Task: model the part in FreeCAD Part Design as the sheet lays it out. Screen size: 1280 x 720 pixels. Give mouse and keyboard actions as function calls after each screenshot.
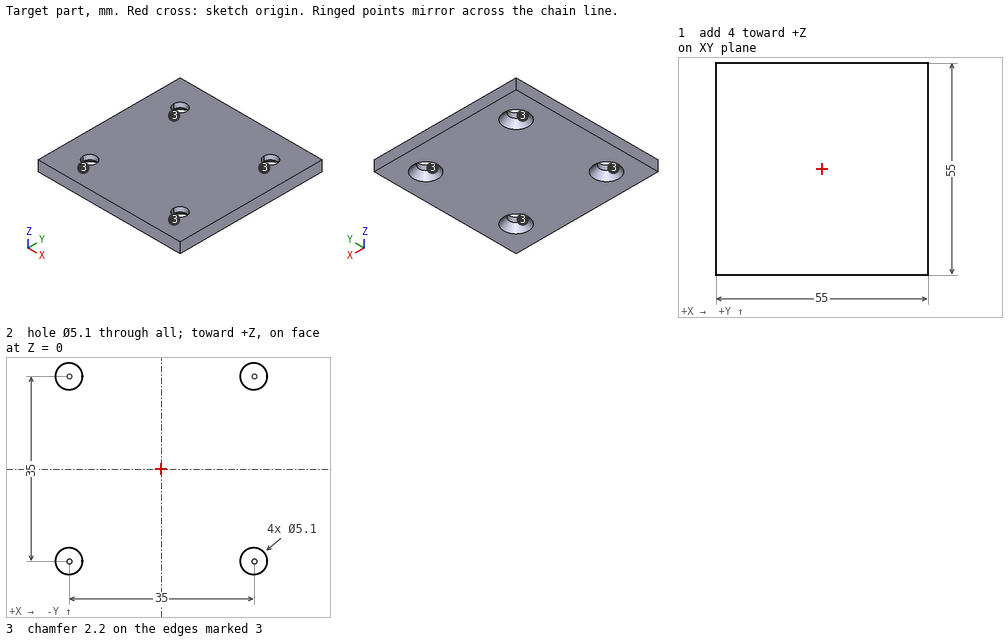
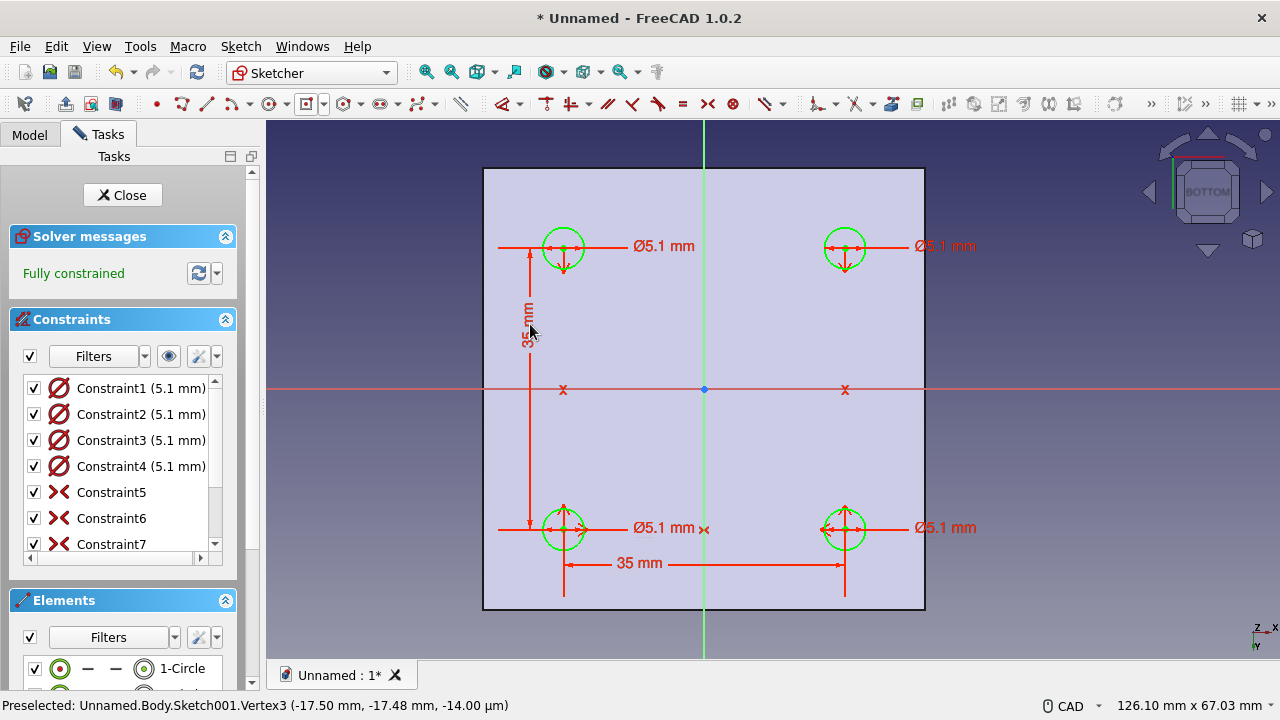
click(123, 195)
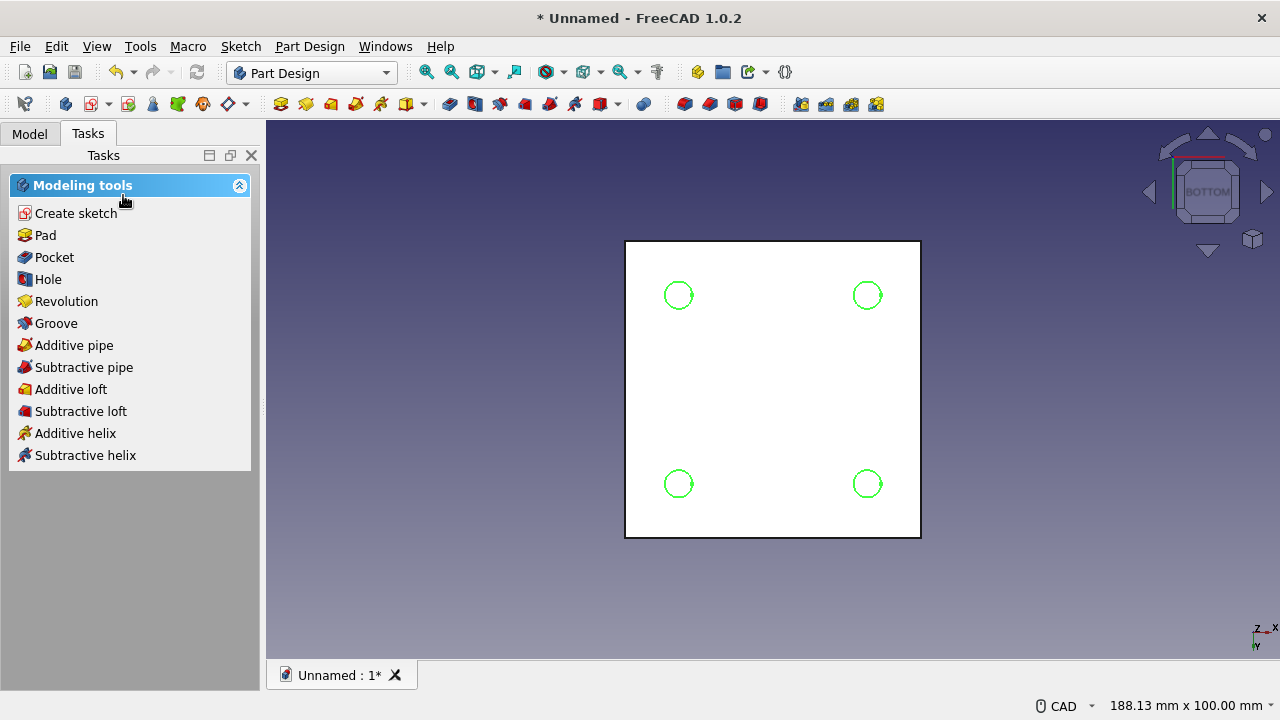
click(475, 104)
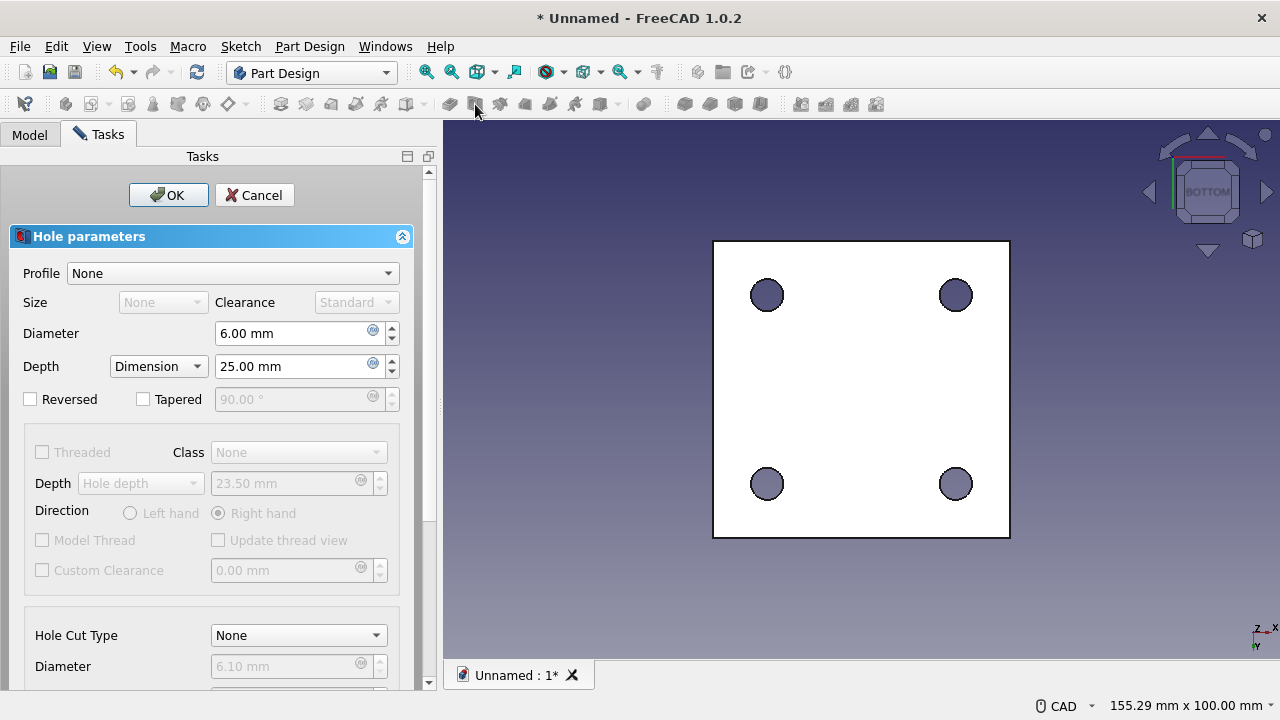
triple_click(300, 334)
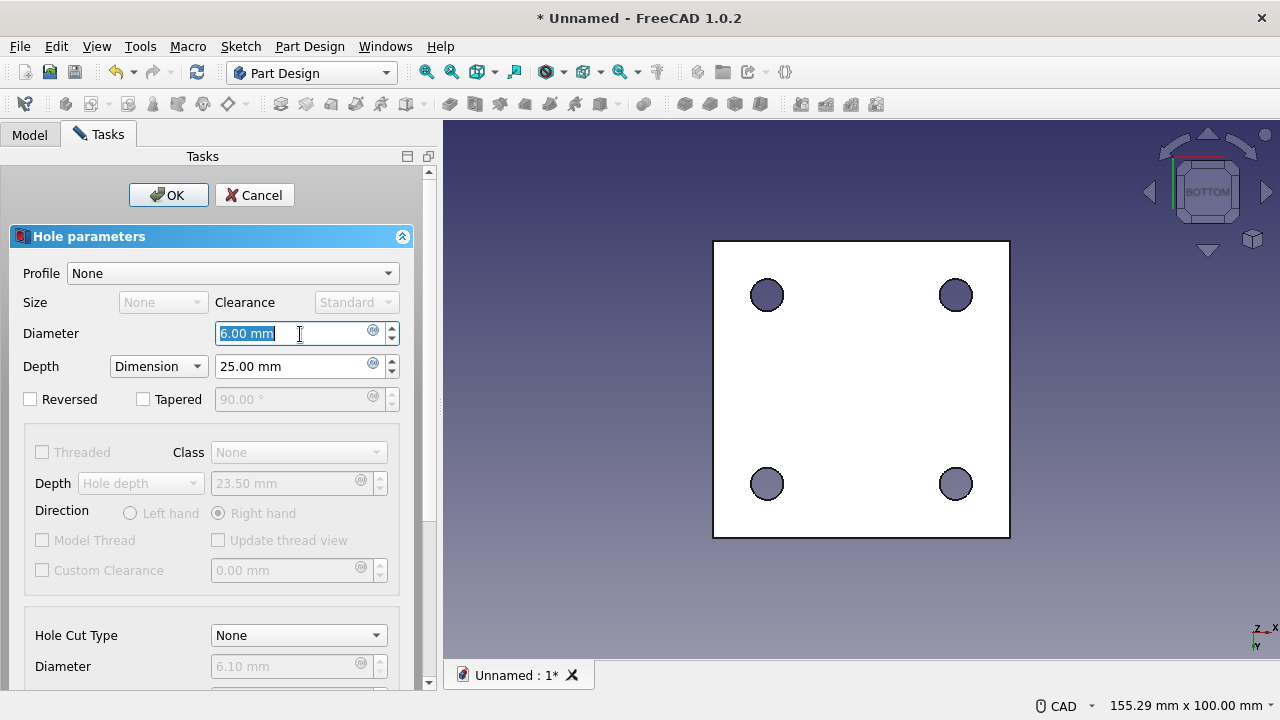
text(5.1)
key(Tab)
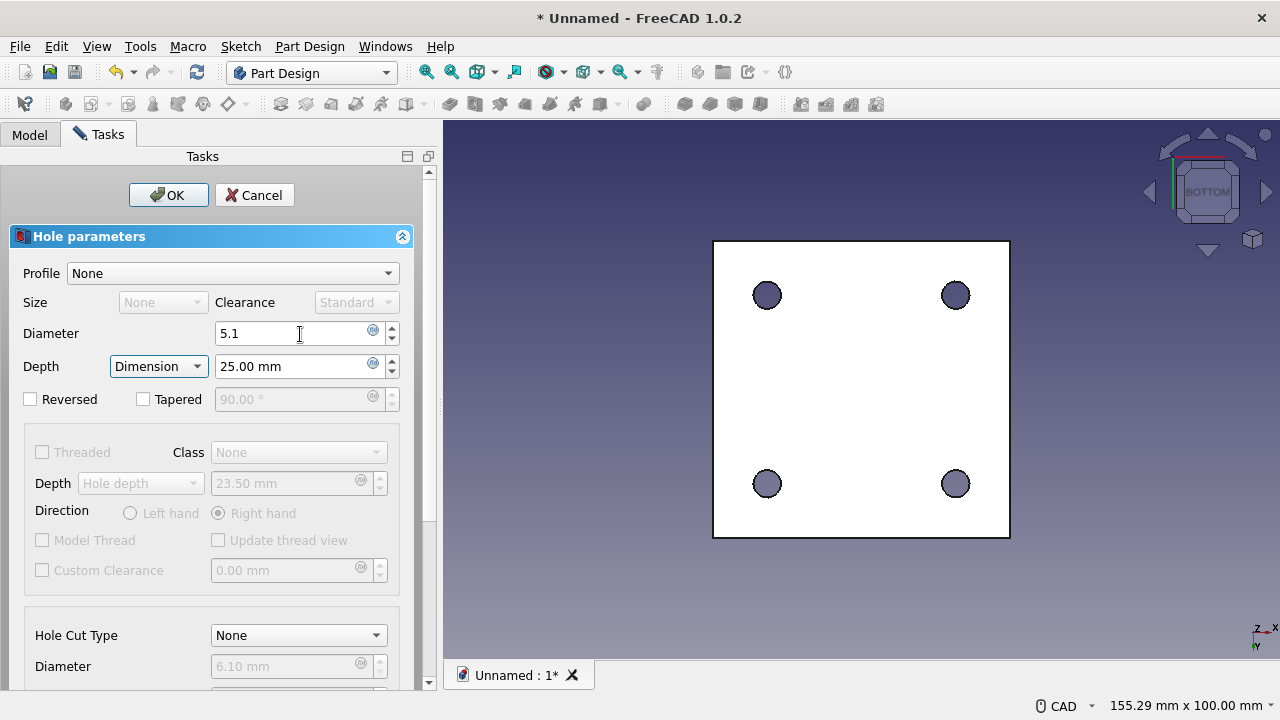
click(160, 366)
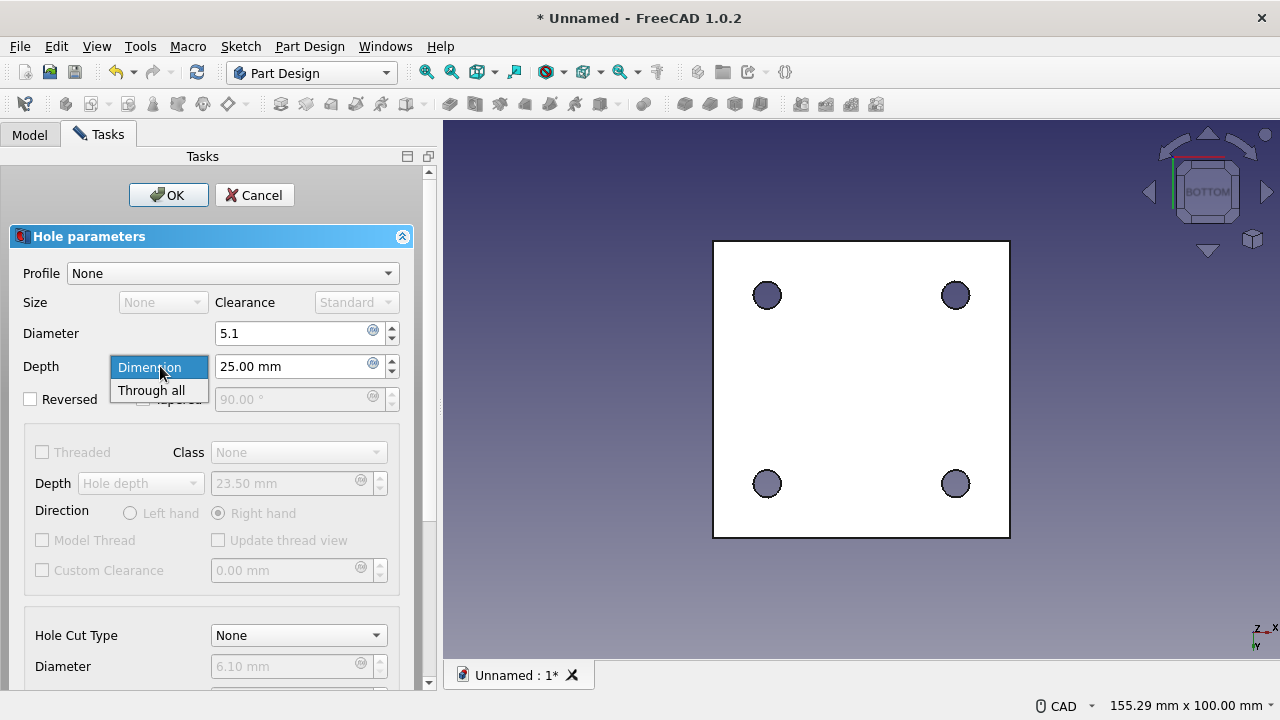
click(158, 390)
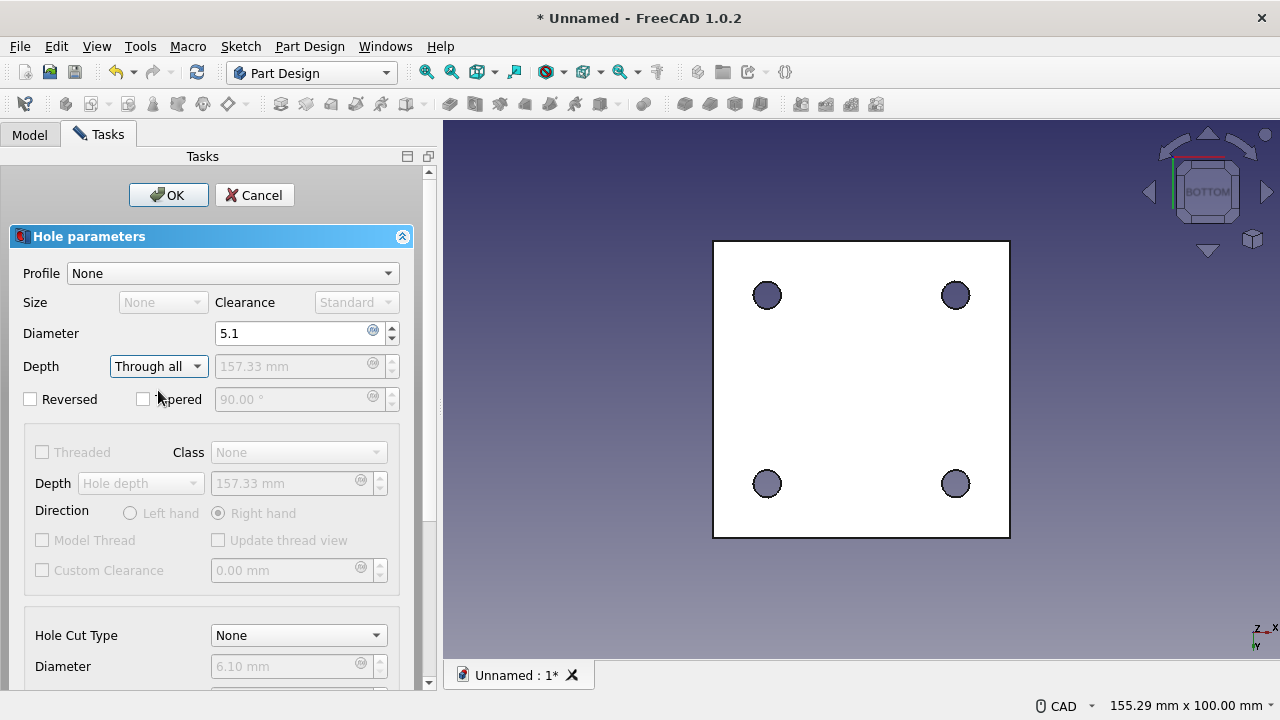
click(169, 195)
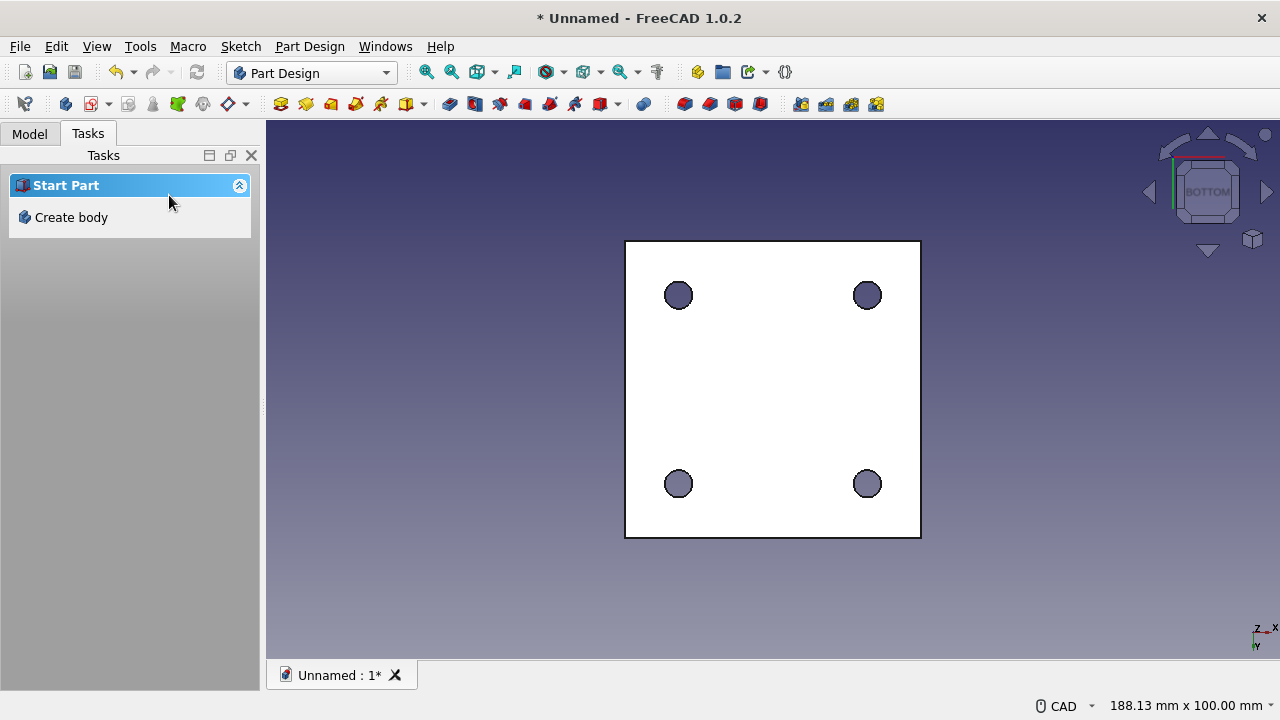
click(881, 294)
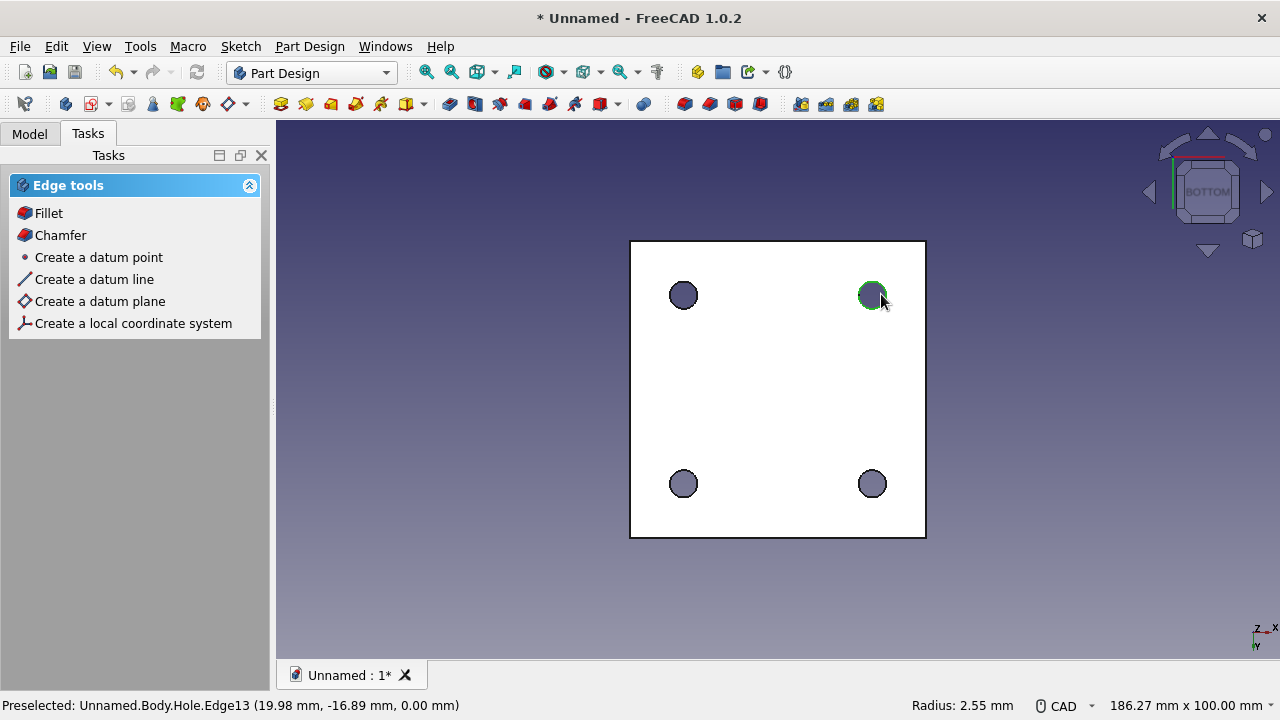
click(697, 294, ctrl)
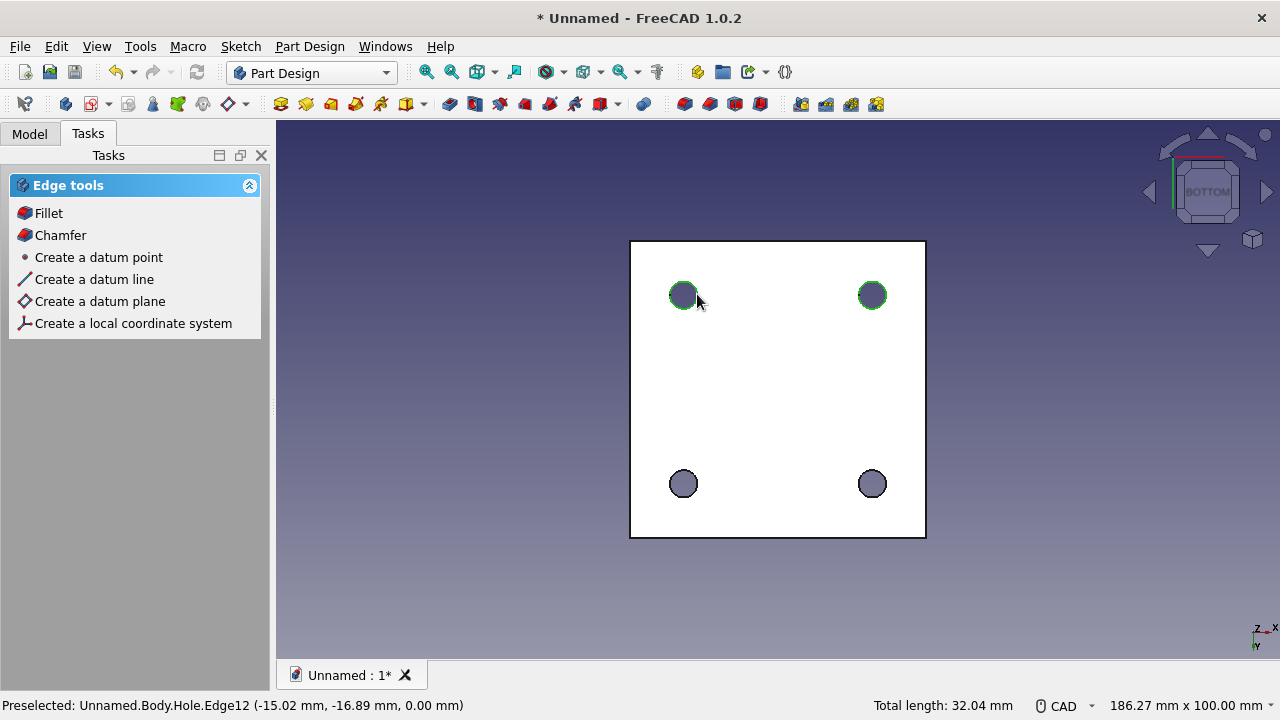
click(697, 483, ctrl)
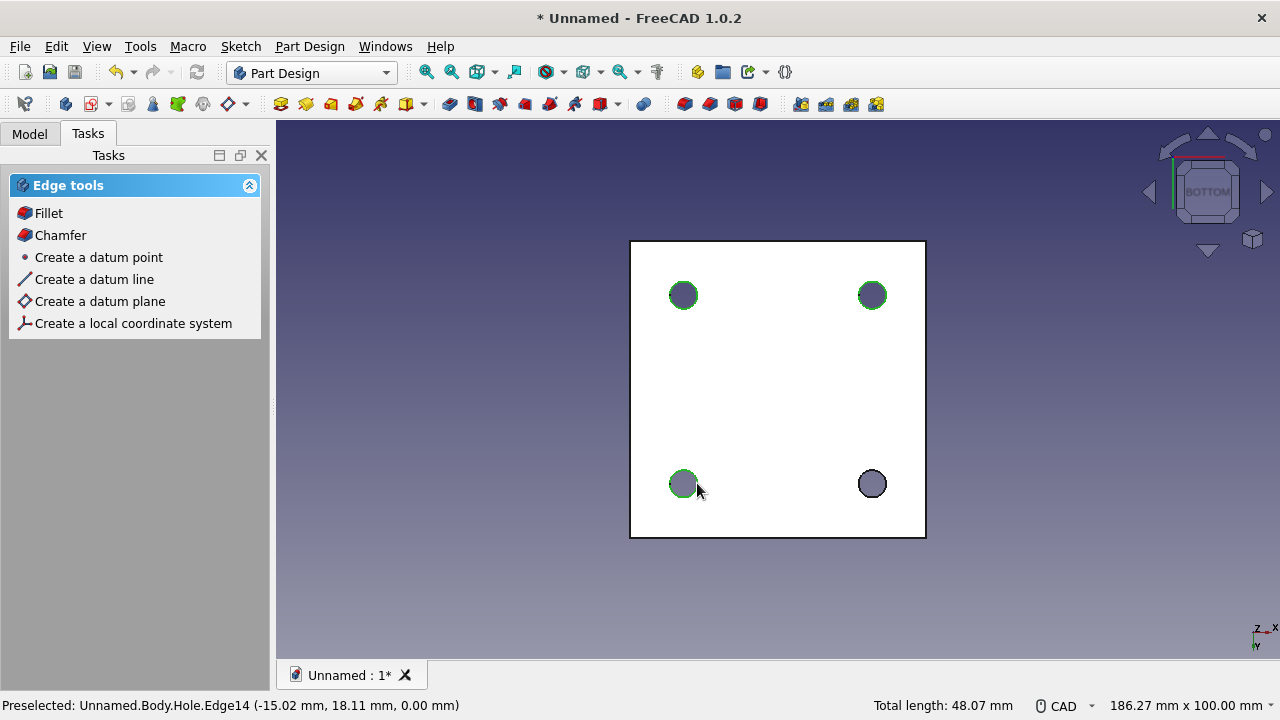
click(886, 483, ctrl)